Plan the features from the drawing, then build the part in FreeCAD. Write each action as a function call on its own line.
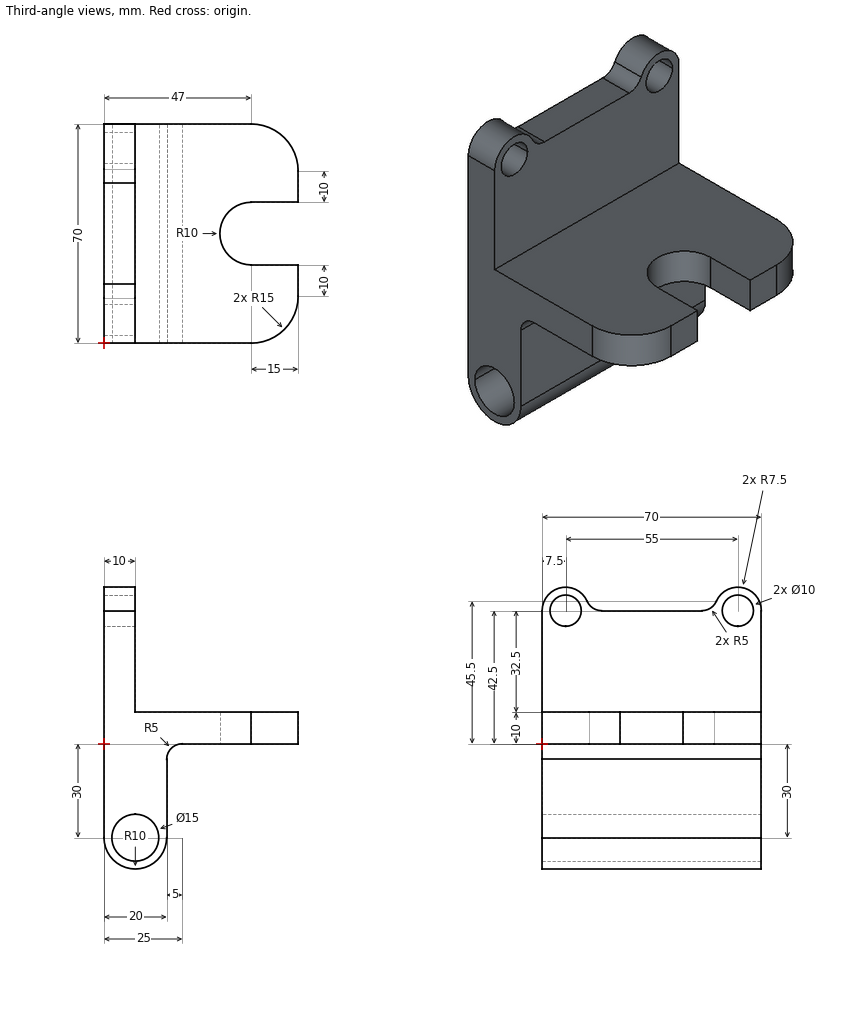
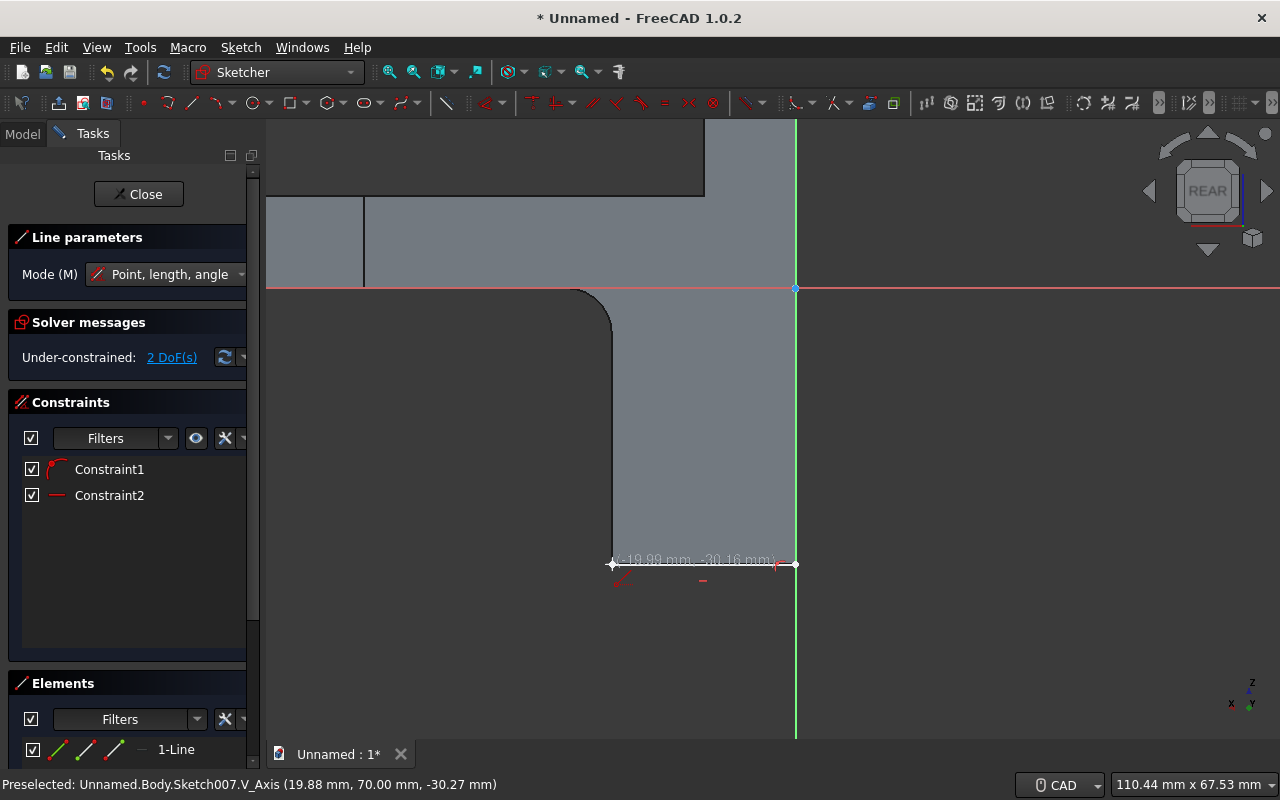
click(216, 104)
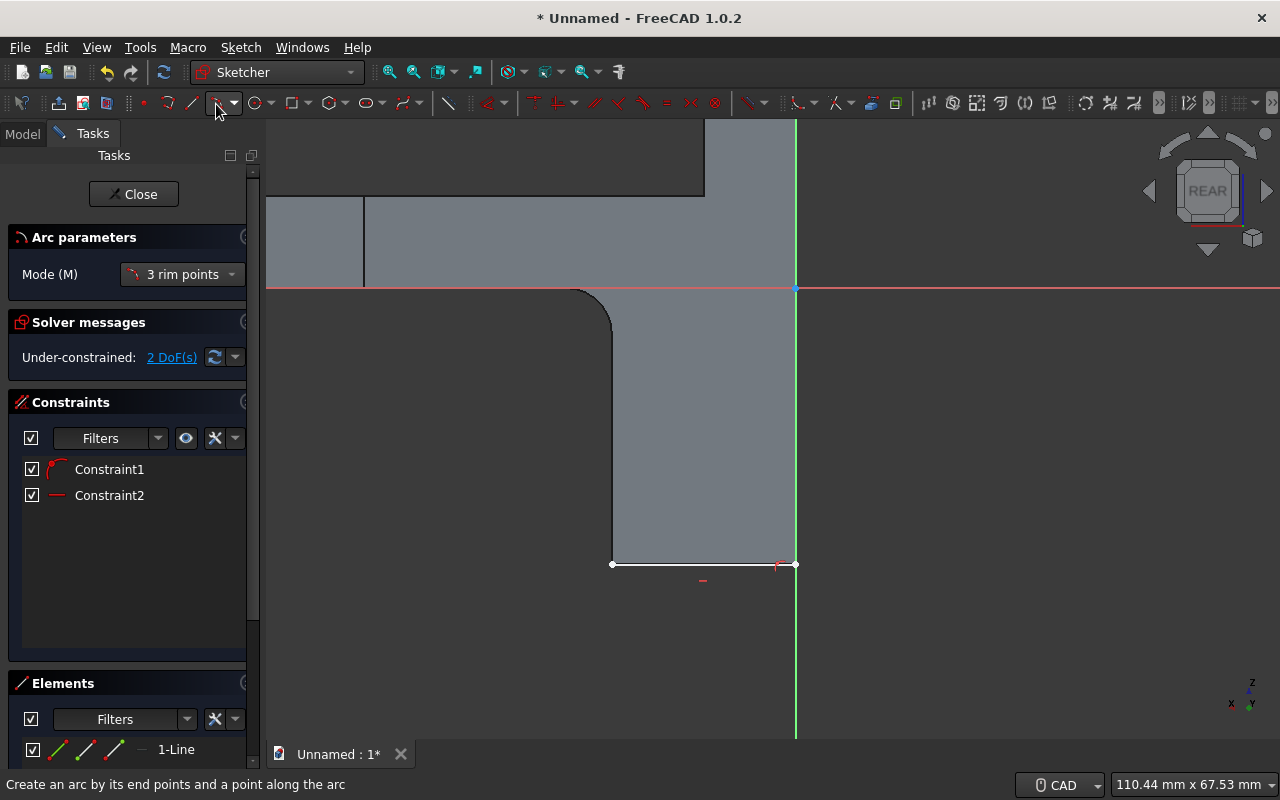
click(612, 565)
click(796, 565)
click(704, 655)
key(Escape)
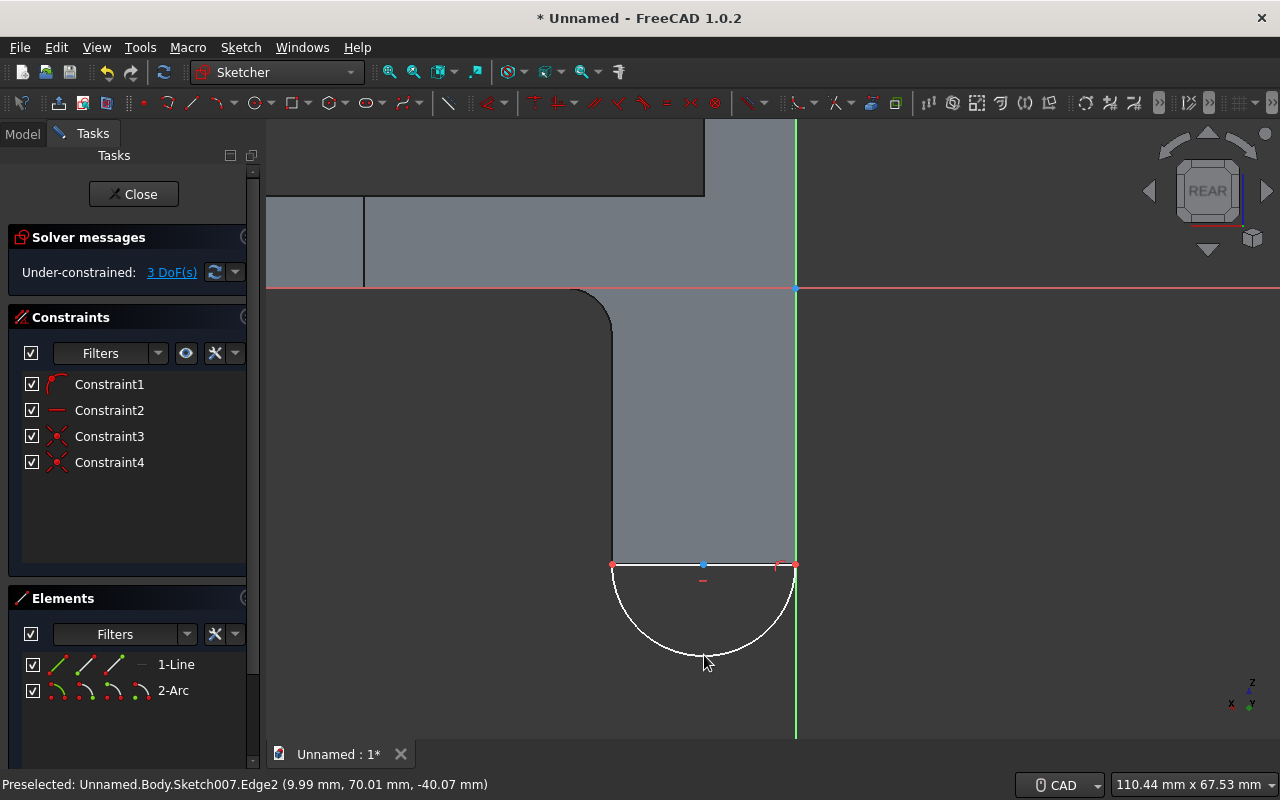
click(488, 104)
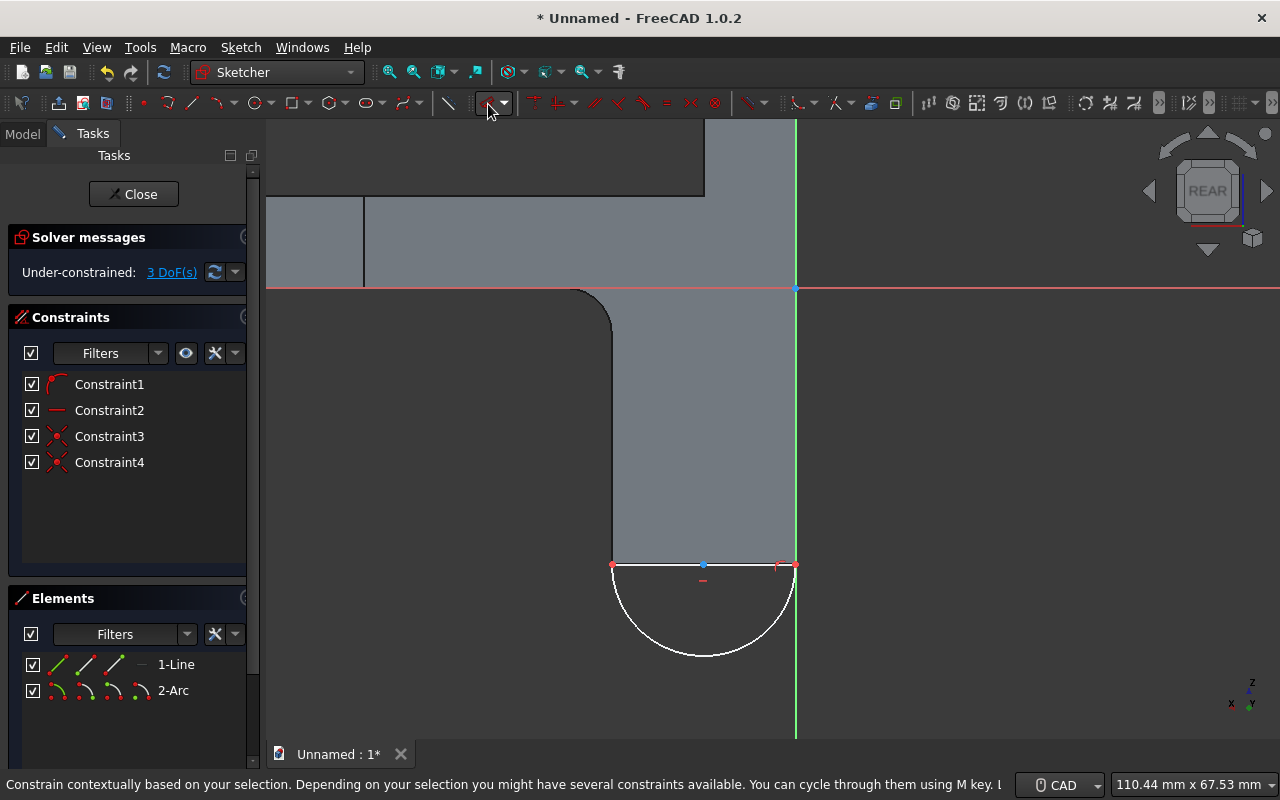
click(650, 639)
click(631, 665)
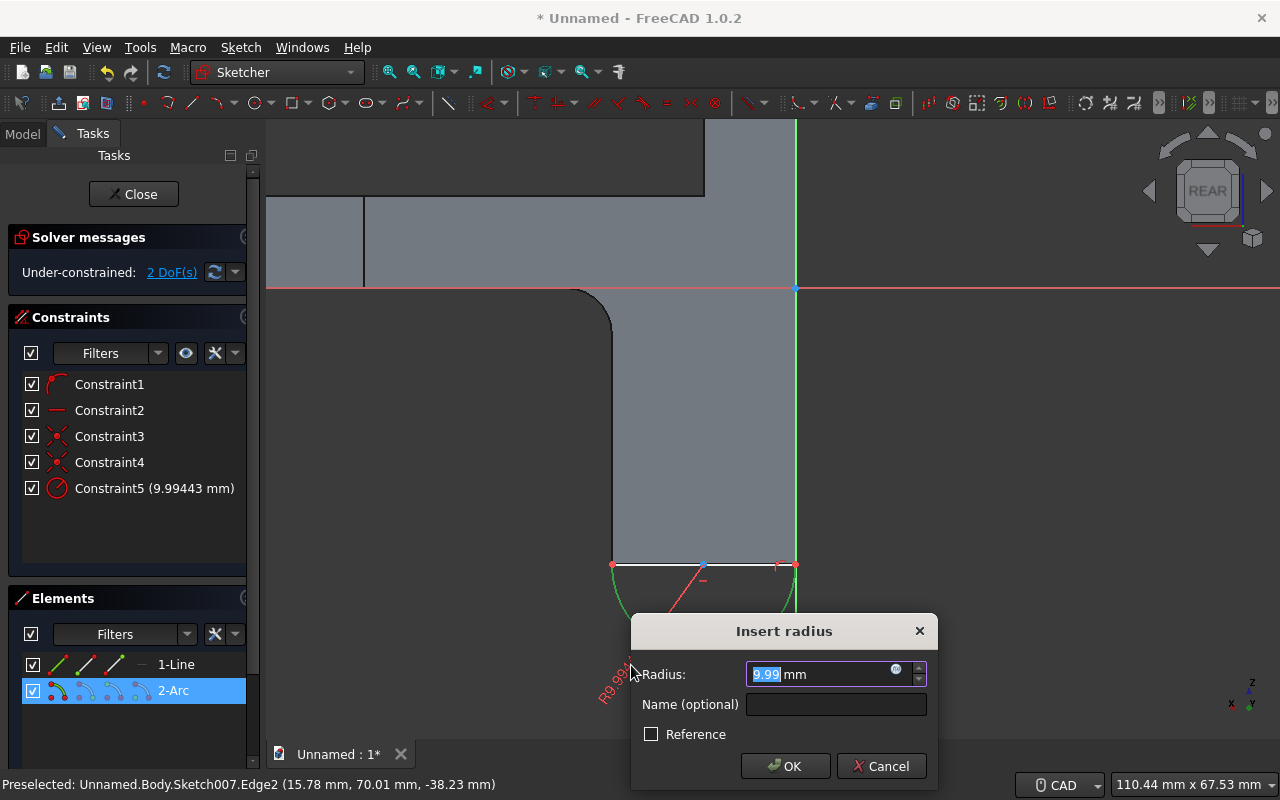
text(10)
key(Return)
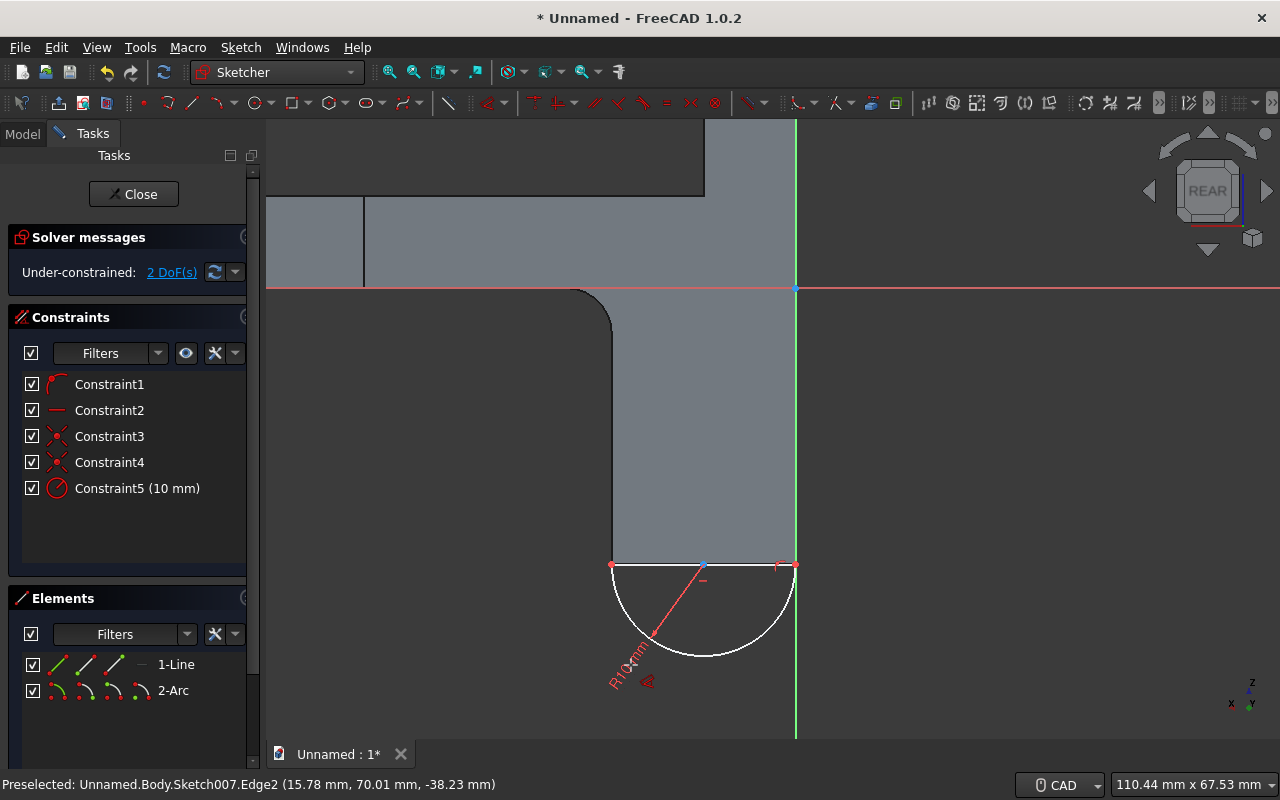
click(796, 565)
click(830, 427)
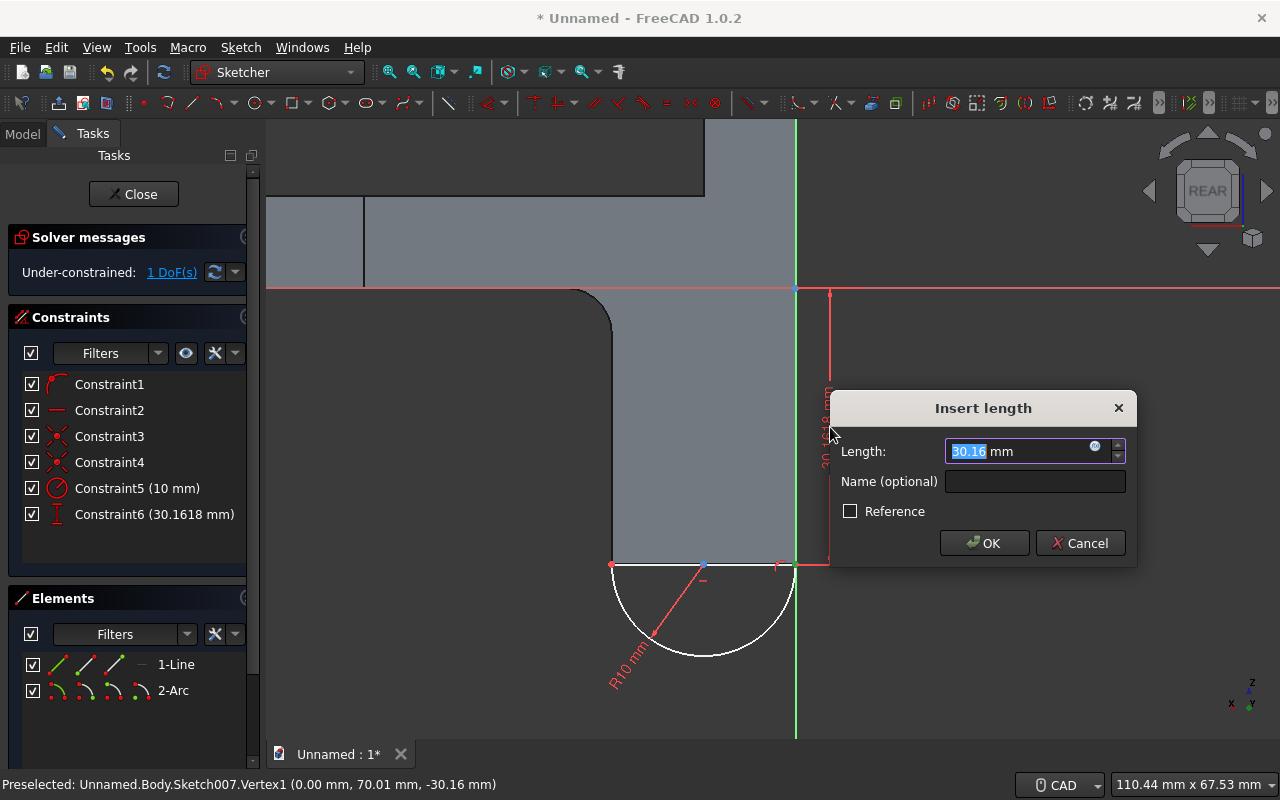
text(30)
key(Return)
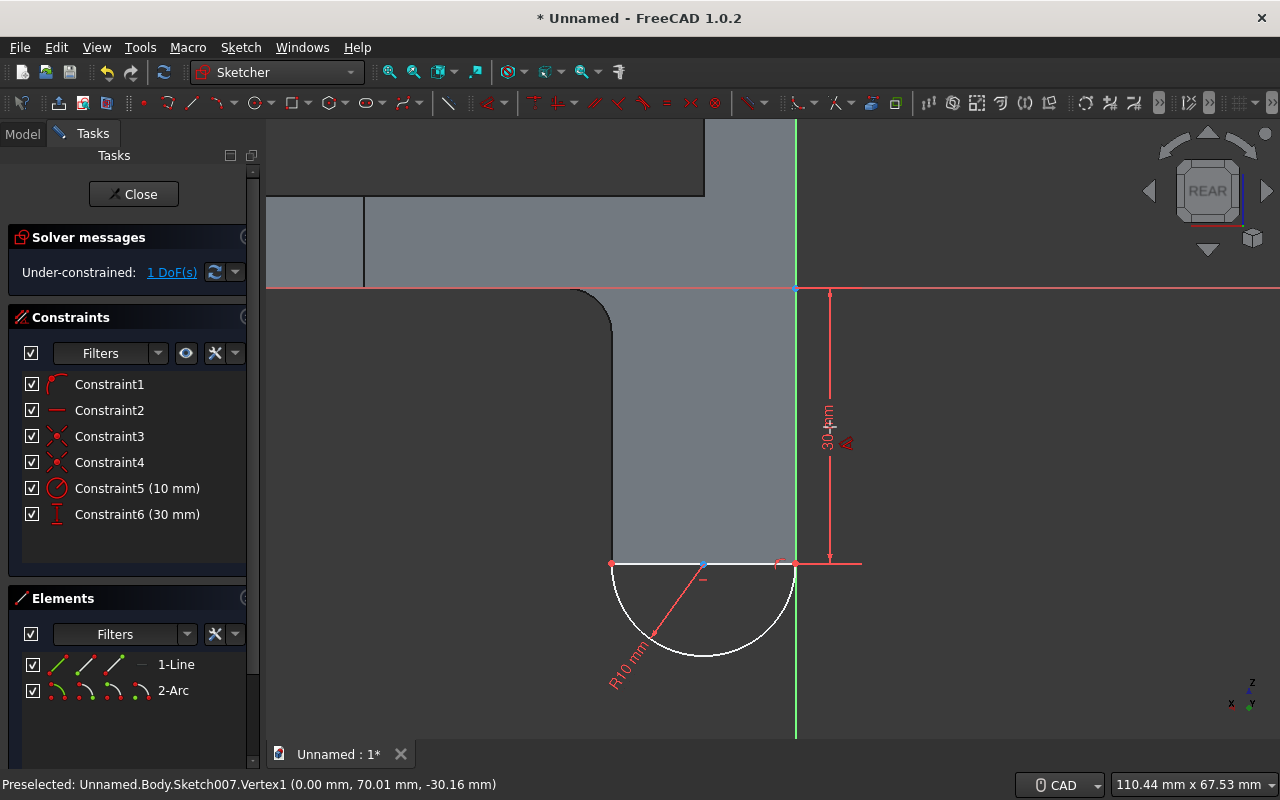
click(704, 564)
click(830, 363)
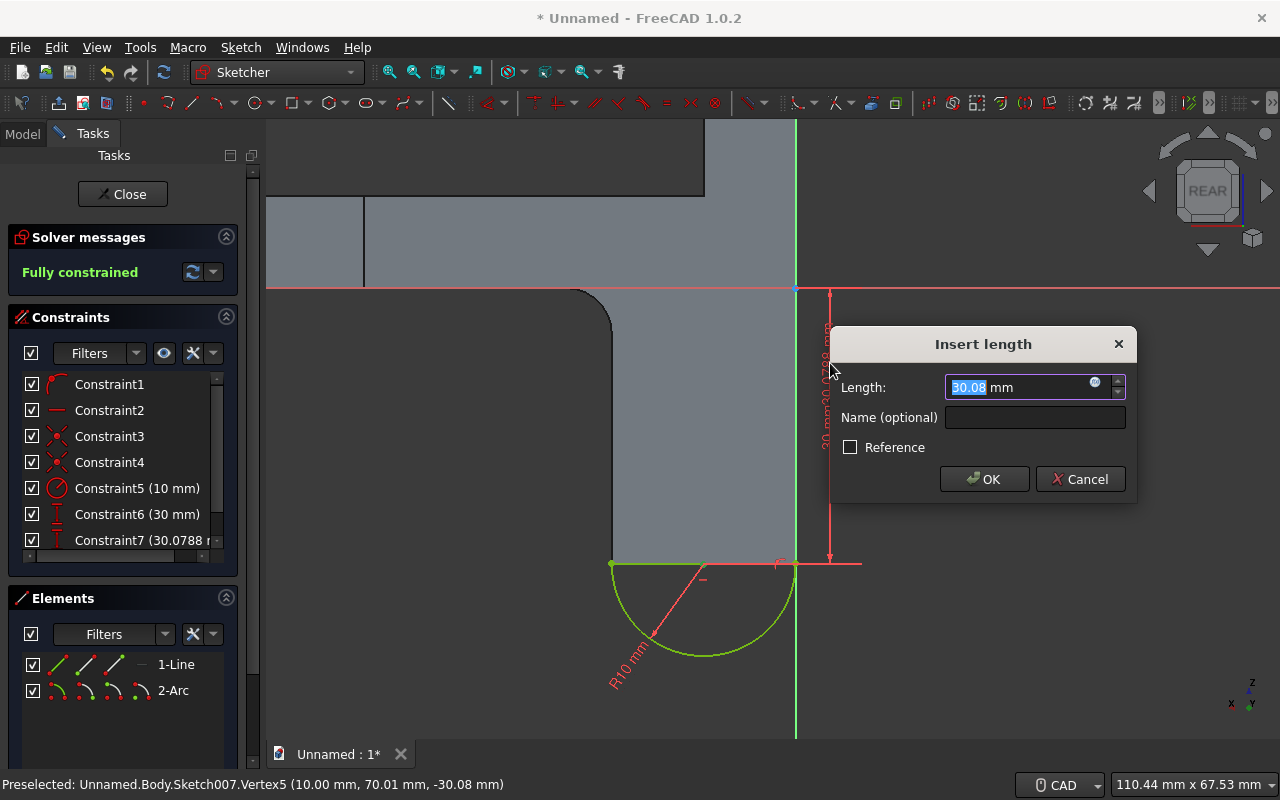
text(30)
key(Return)
key(Escape)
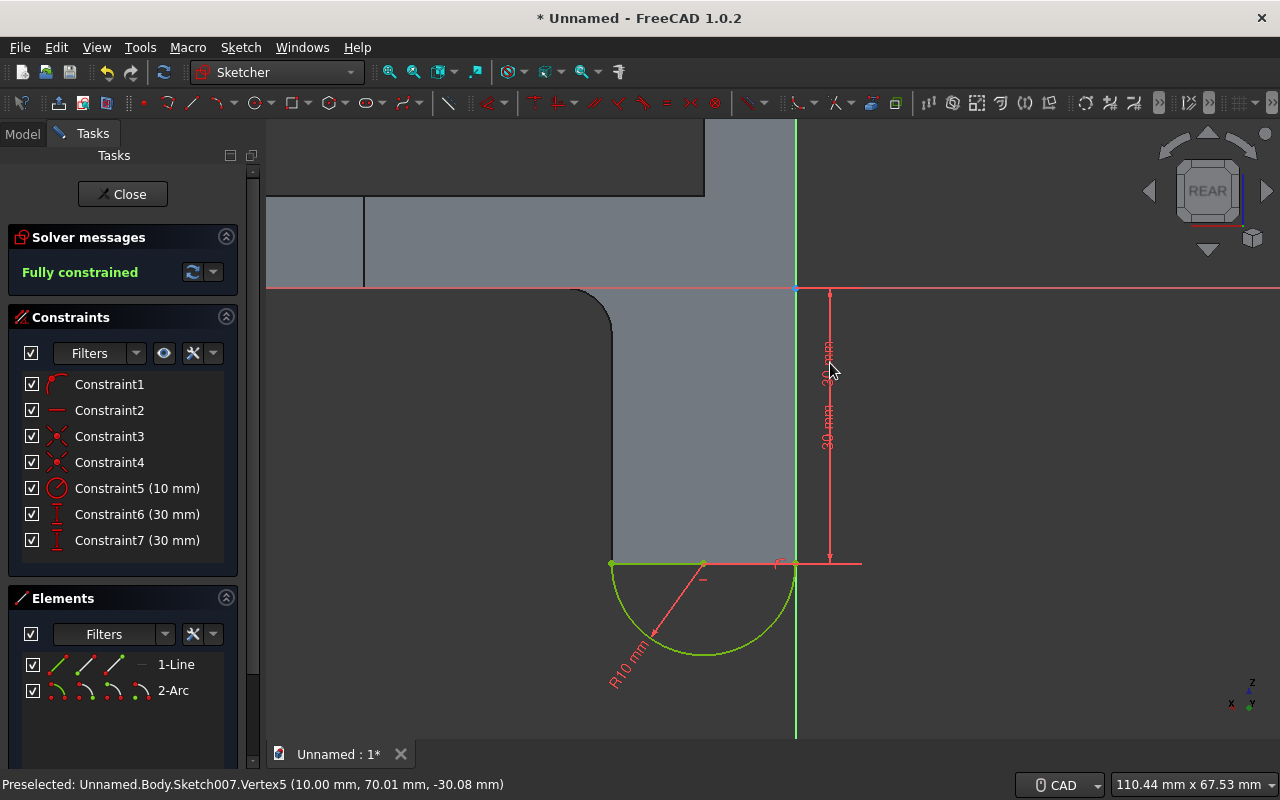
click(123, 194)